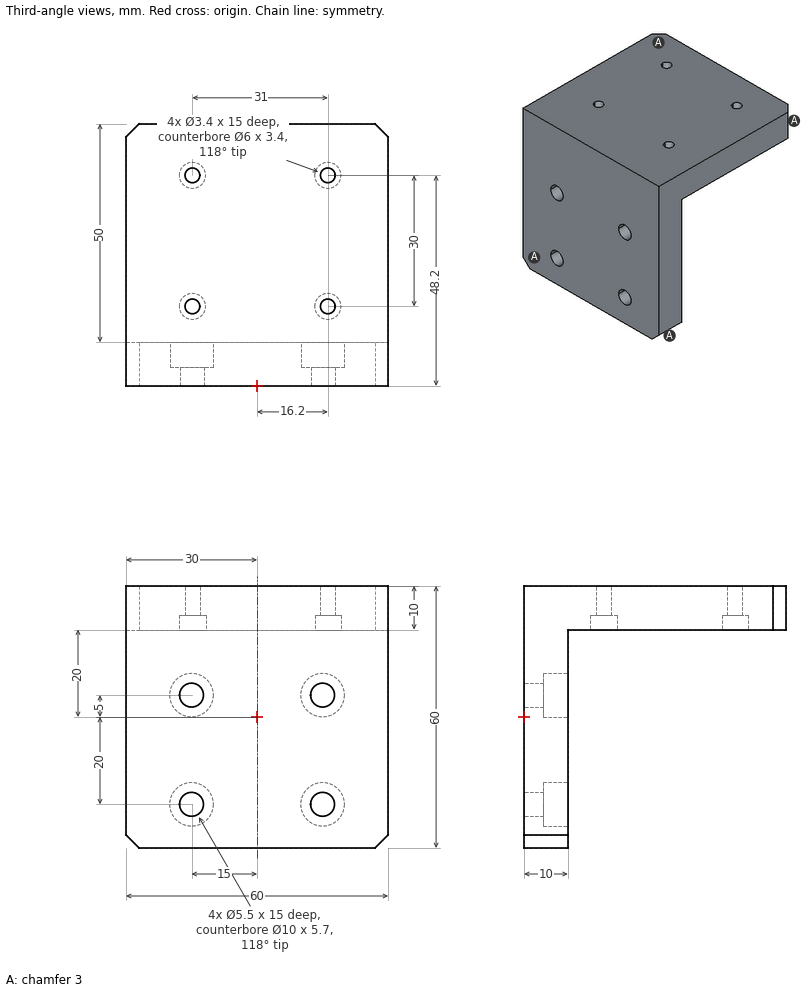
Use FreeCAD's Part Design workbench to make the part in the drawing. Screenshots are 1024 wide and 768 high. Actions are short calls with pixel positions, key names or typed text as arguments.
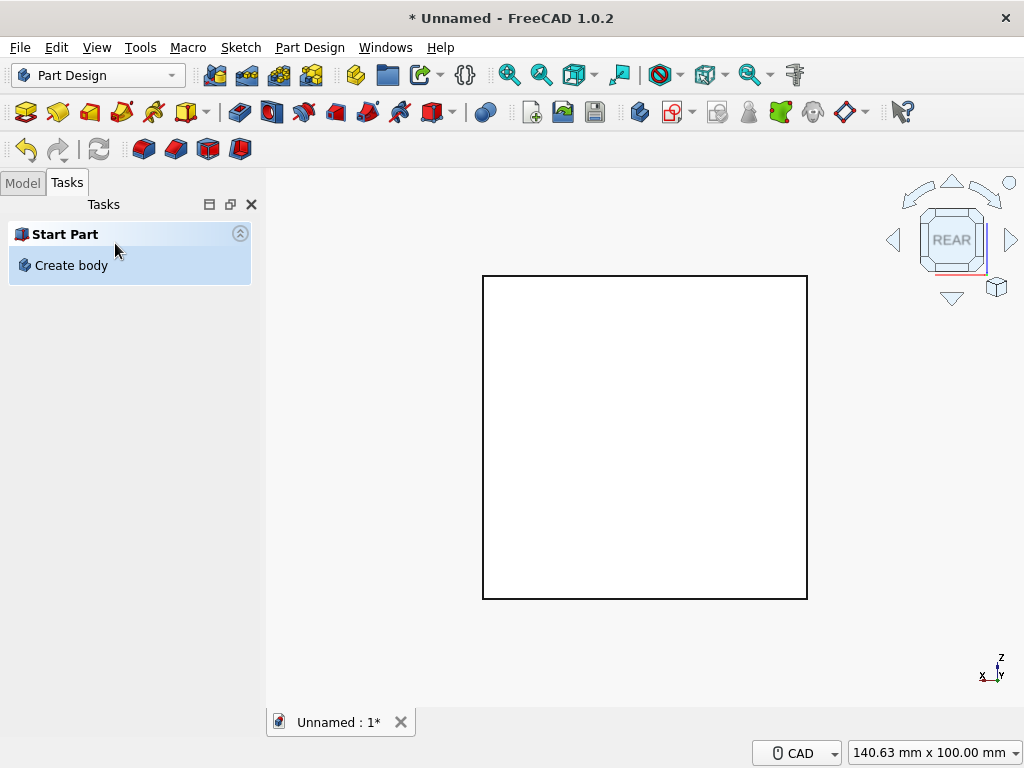
click(645, 436)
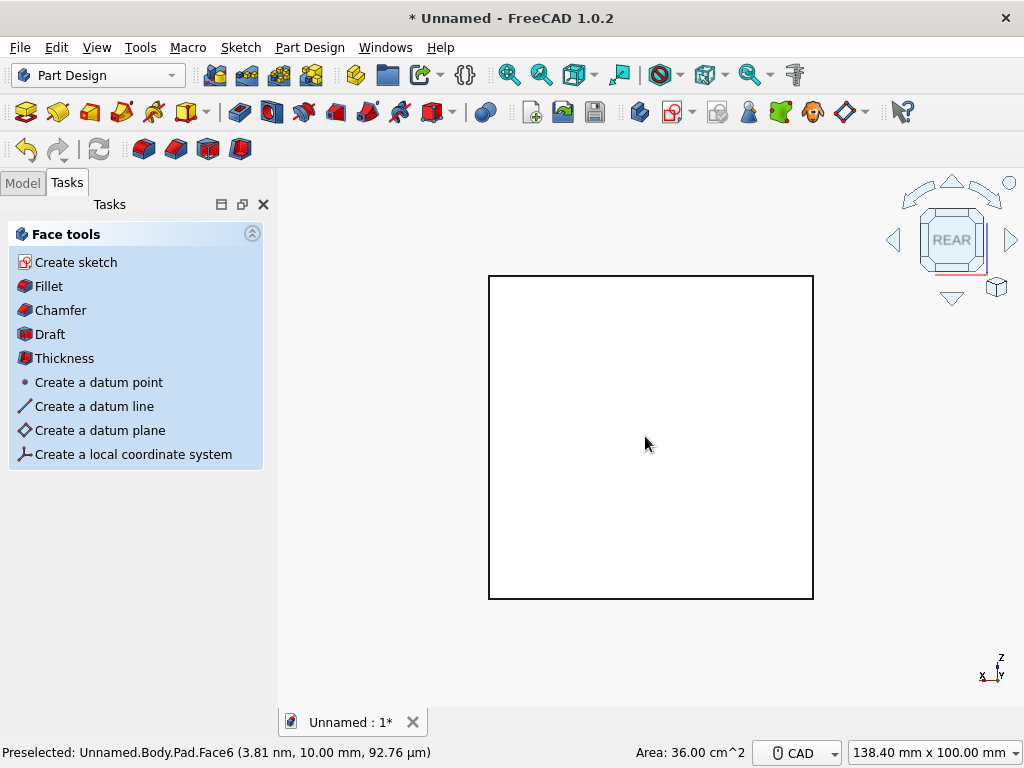
click(672, 112)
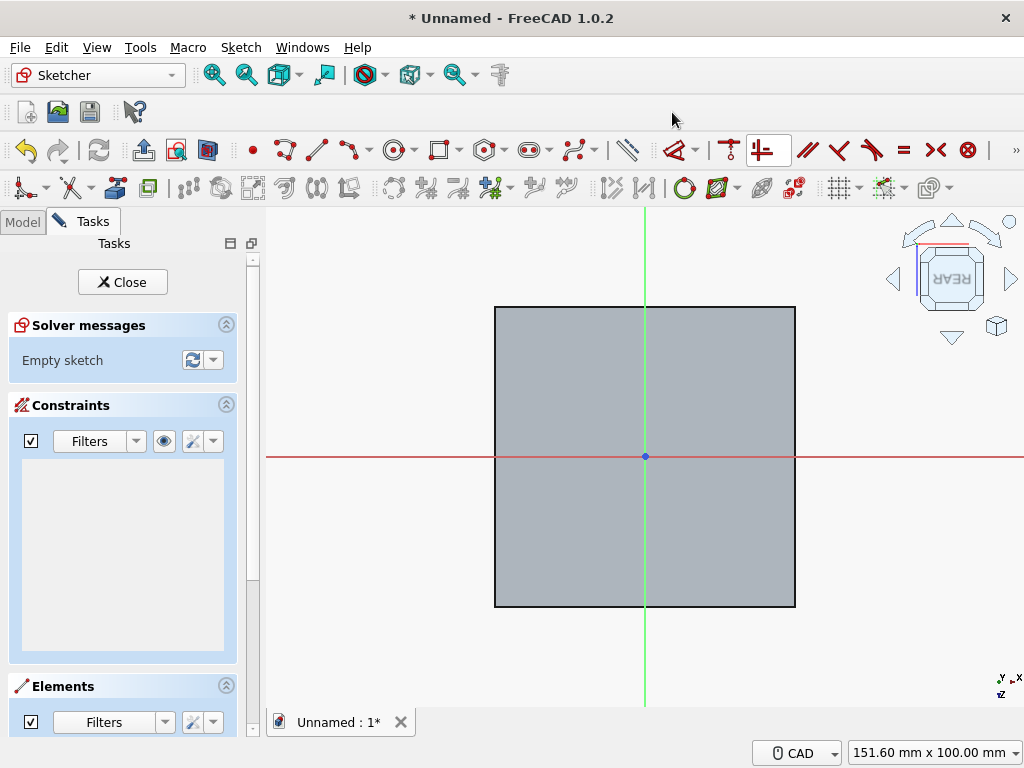
click(440, 150)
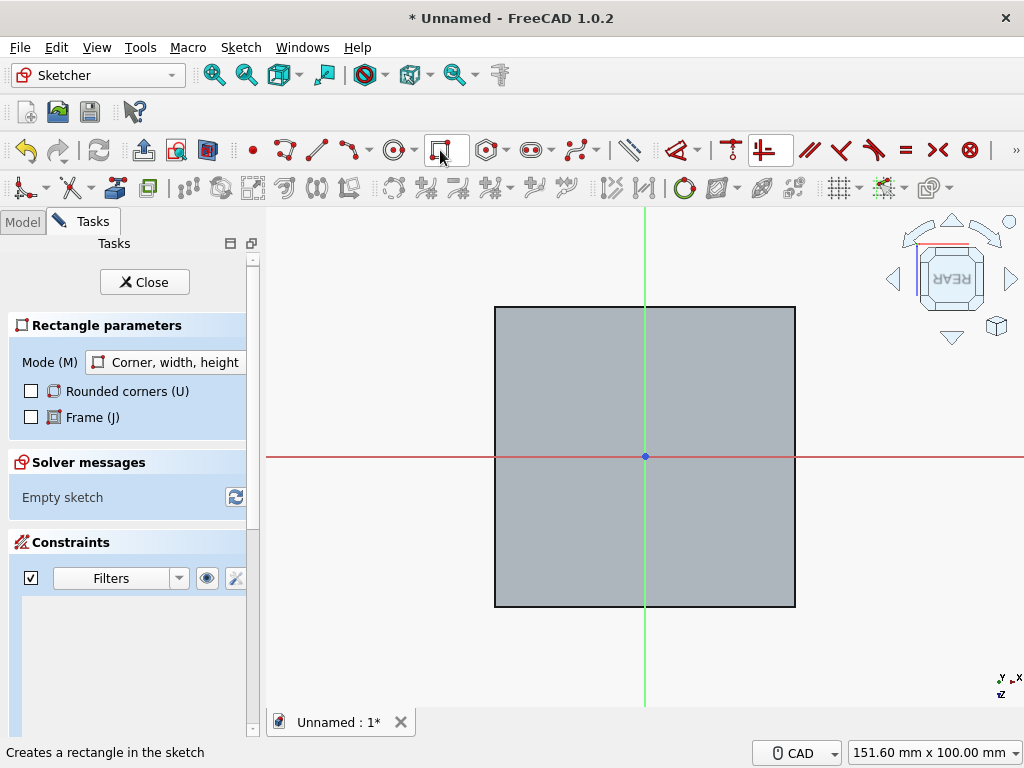
click(495, 557)
move(795, 607)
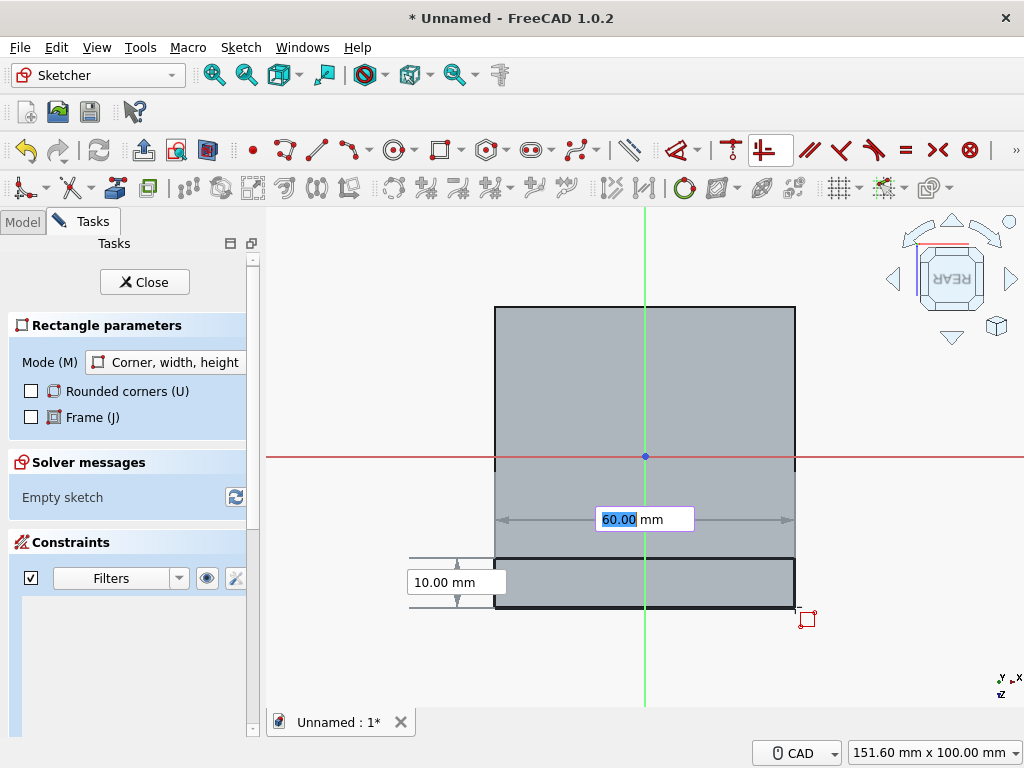
text(60)
key(Tab)
text(10)
key(Return)
key(Escape)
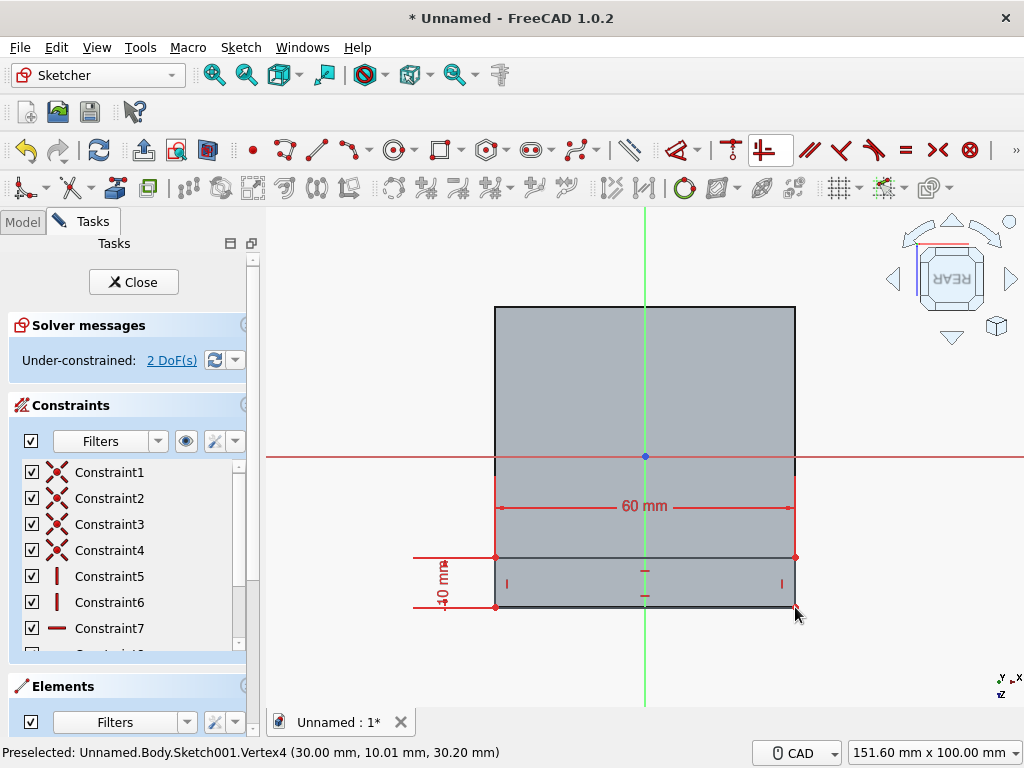
click(676, 150)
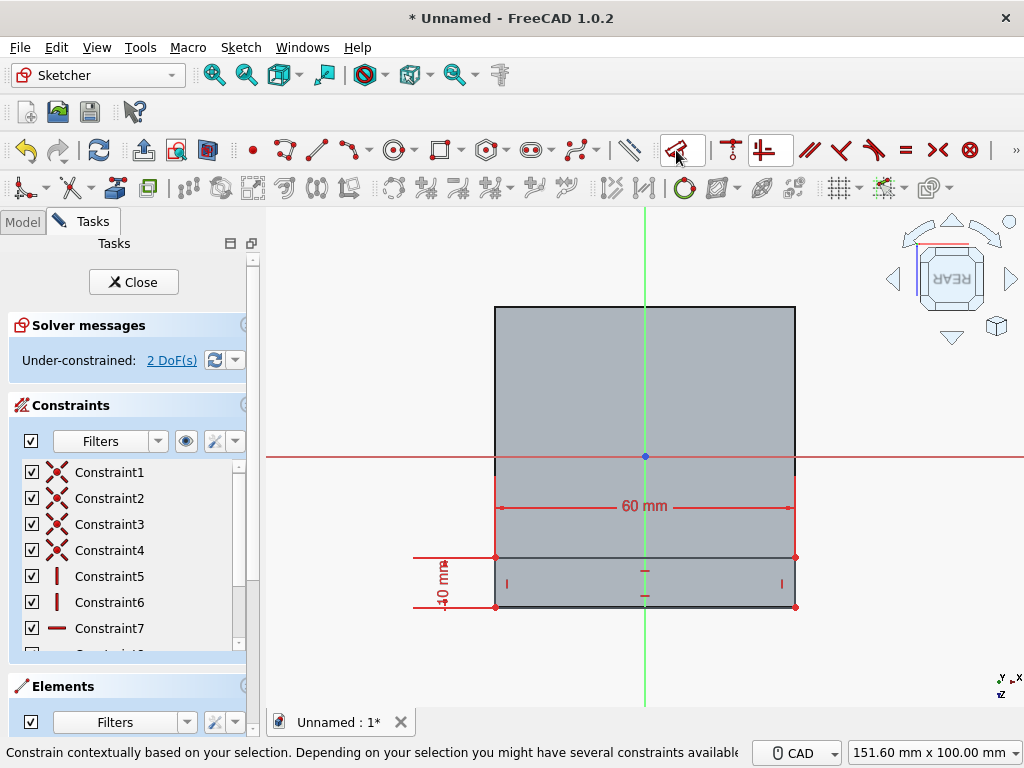
click(495, 558)
click(570, 423)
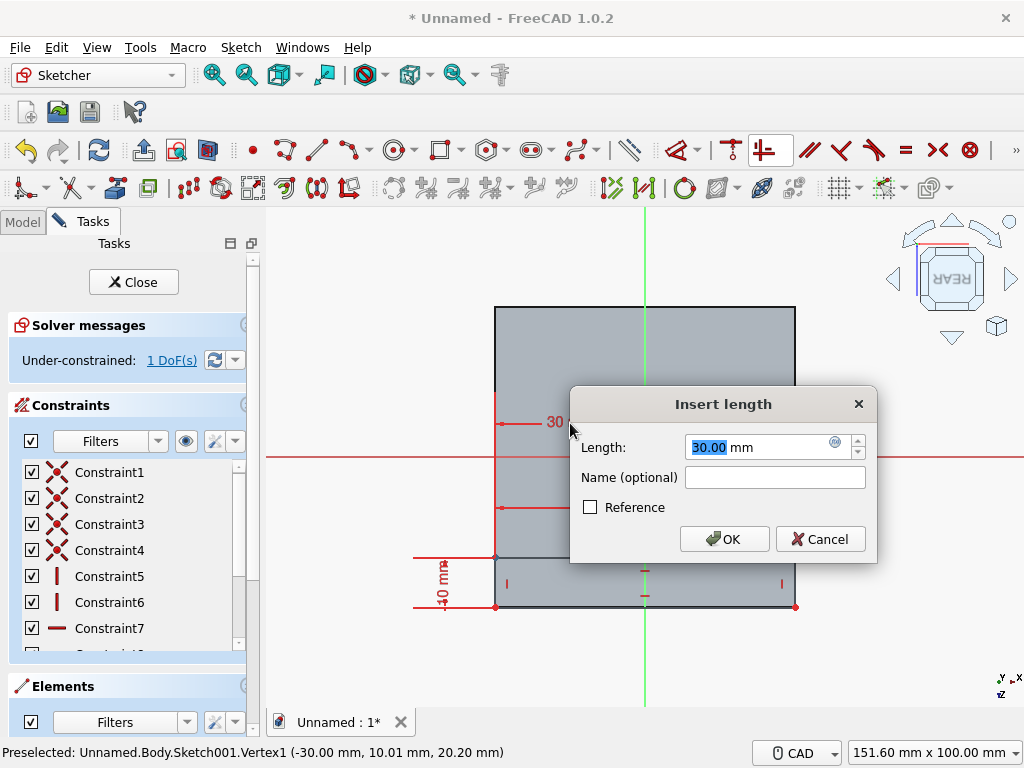
text(30)
key(Return)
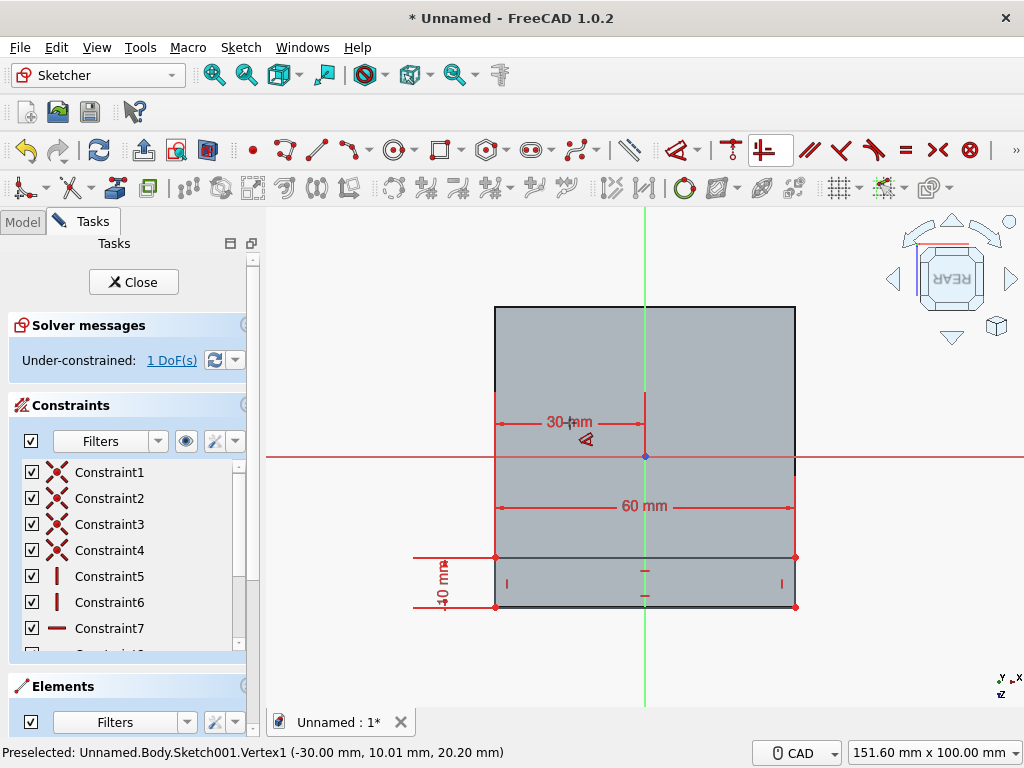
click(495, 558)
click(461, 508)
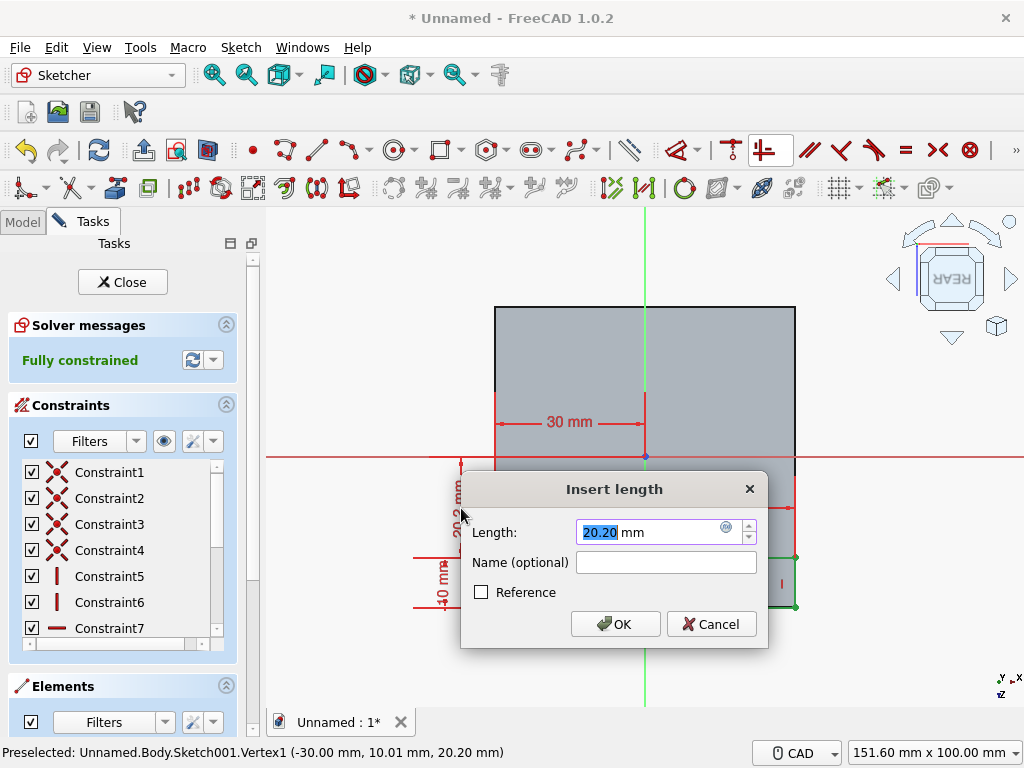
text(20)
key(Return)
key(Escape)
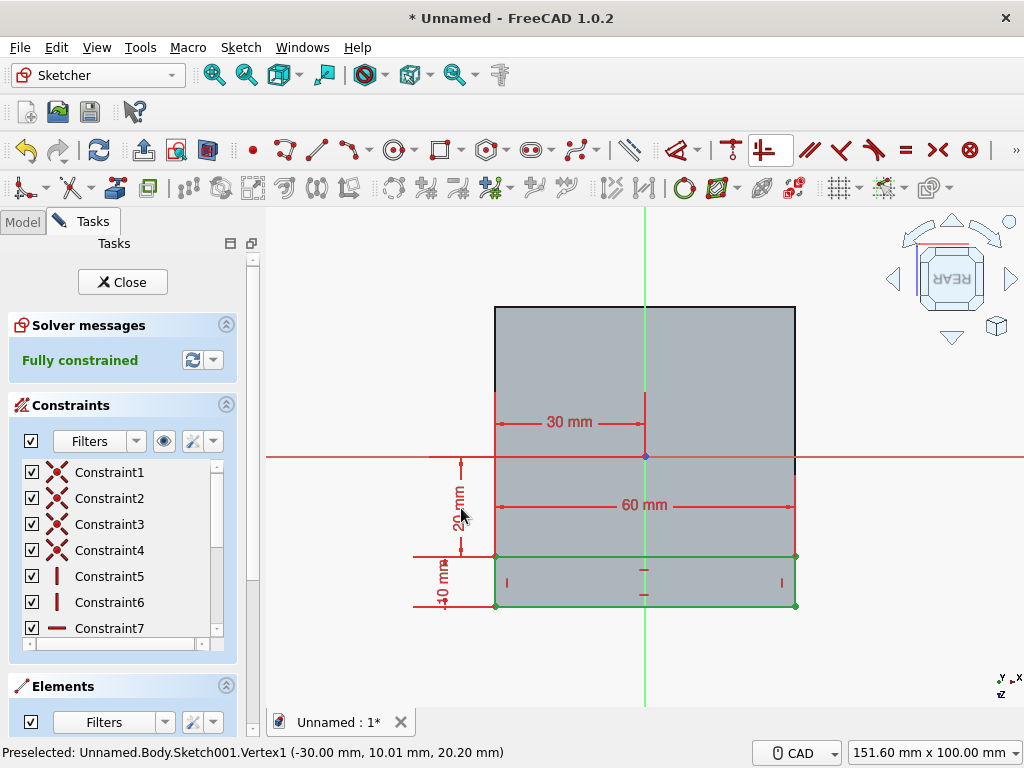
click(123, 282)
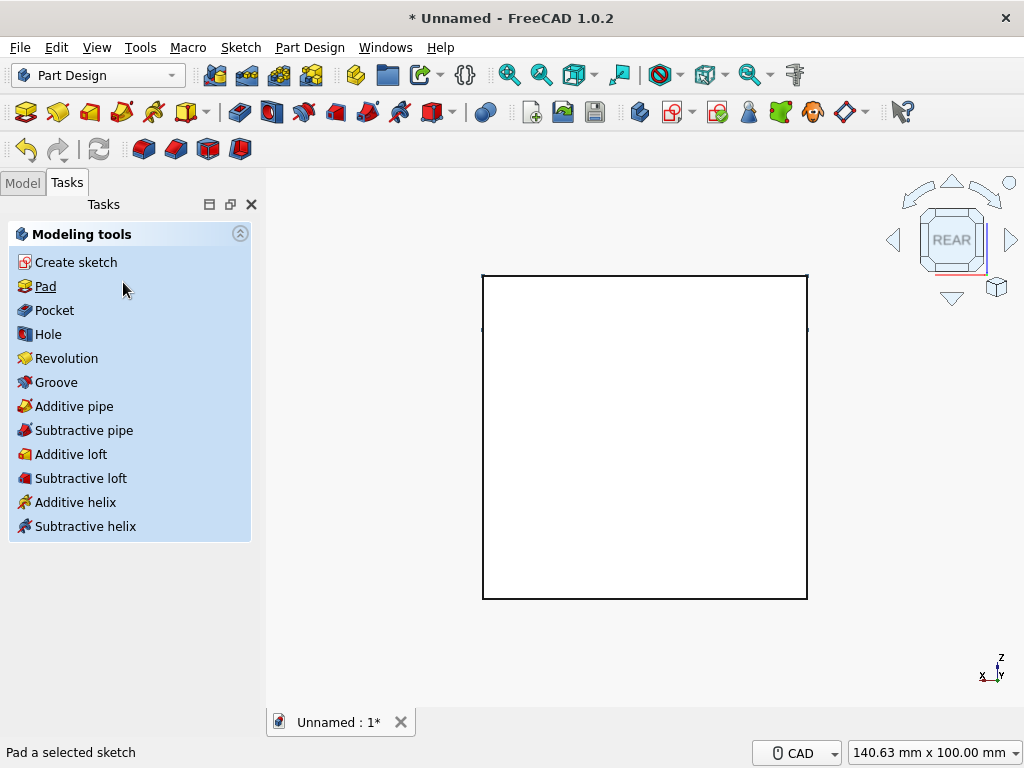
click(26, 112)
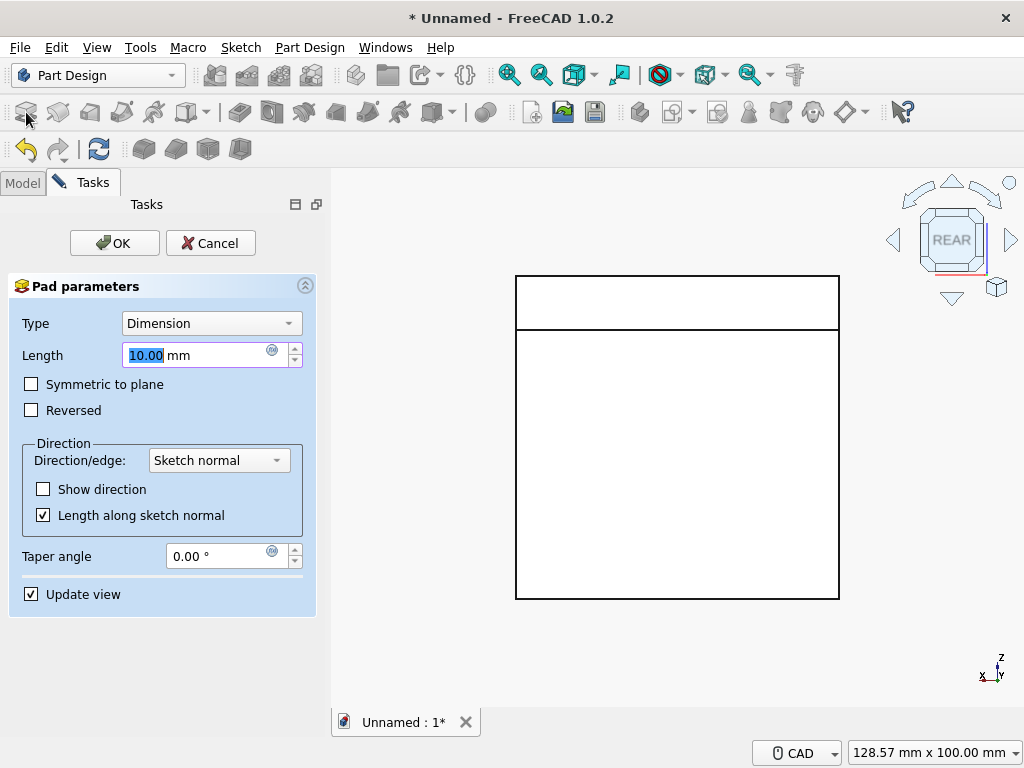
text(50)
key(Tab)